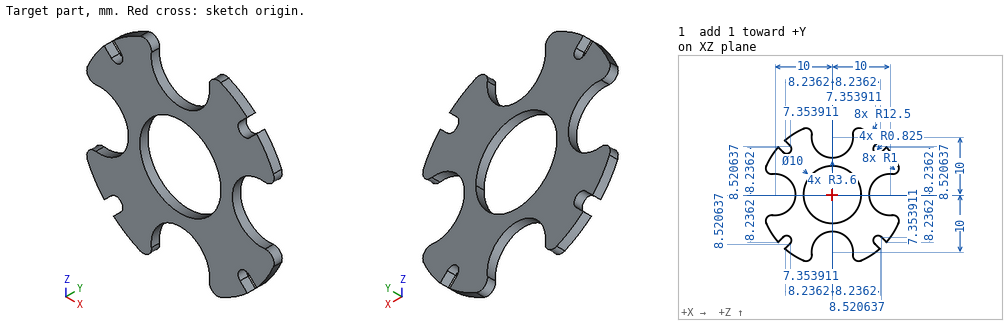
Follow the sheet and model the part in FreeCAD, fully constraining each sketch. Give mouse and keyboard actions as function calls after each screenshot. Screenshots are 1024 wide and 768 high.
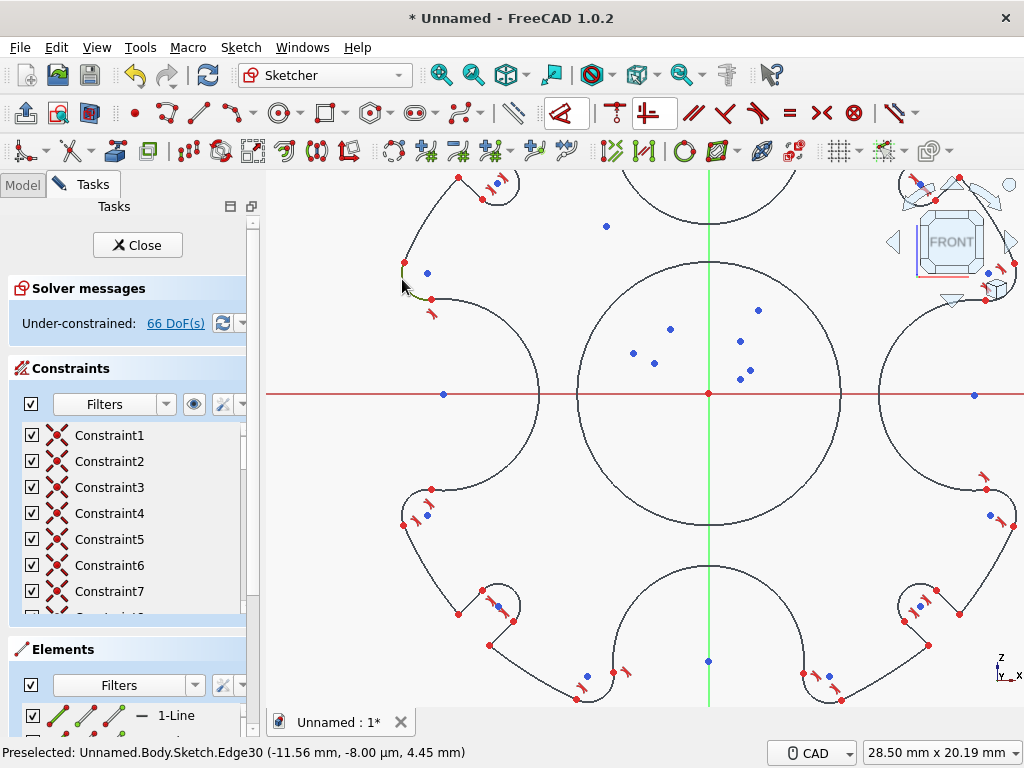
click(439, 201)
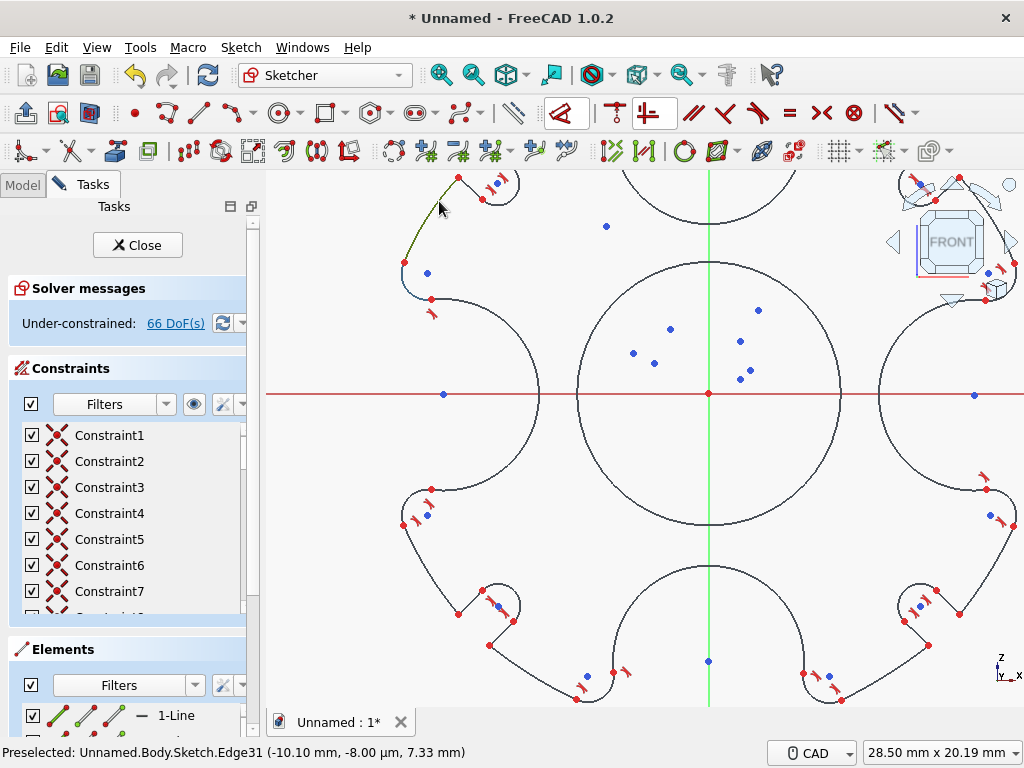
click(758, 114)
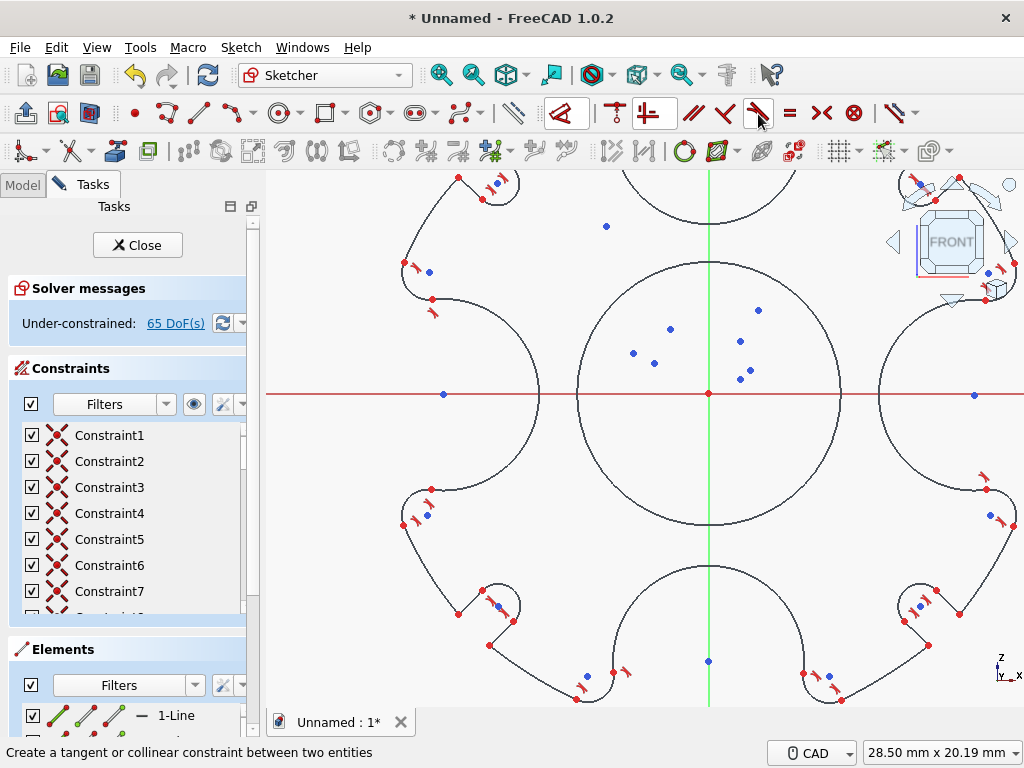
click(802, 300)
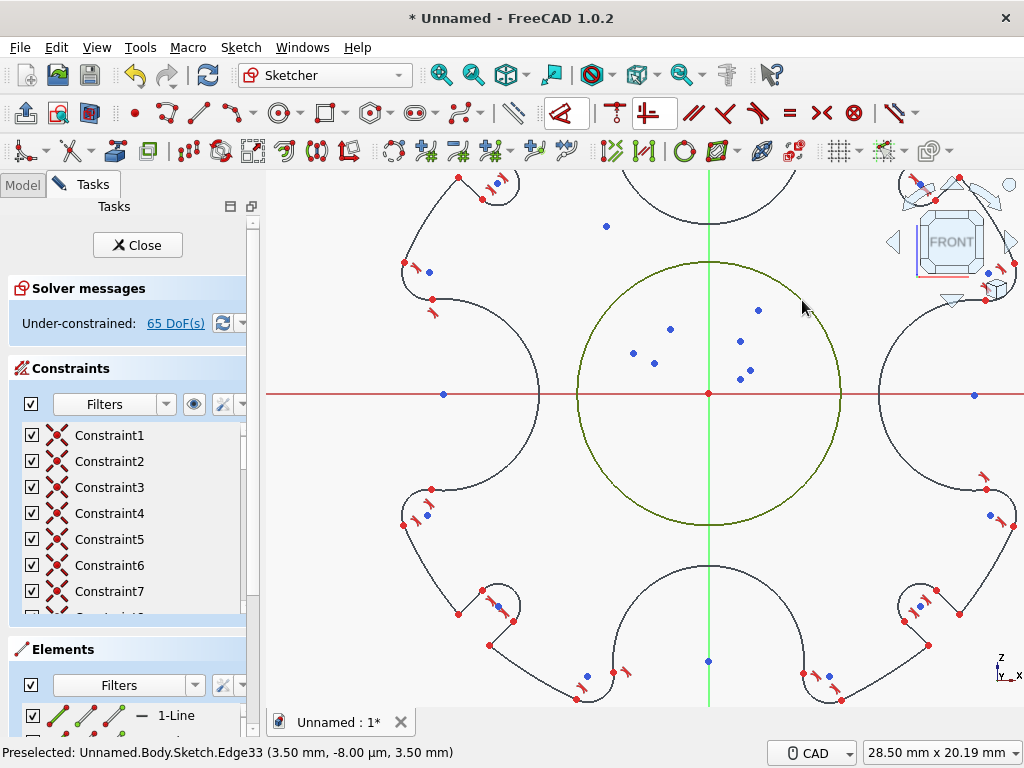
scroll(415, 493, down, 3)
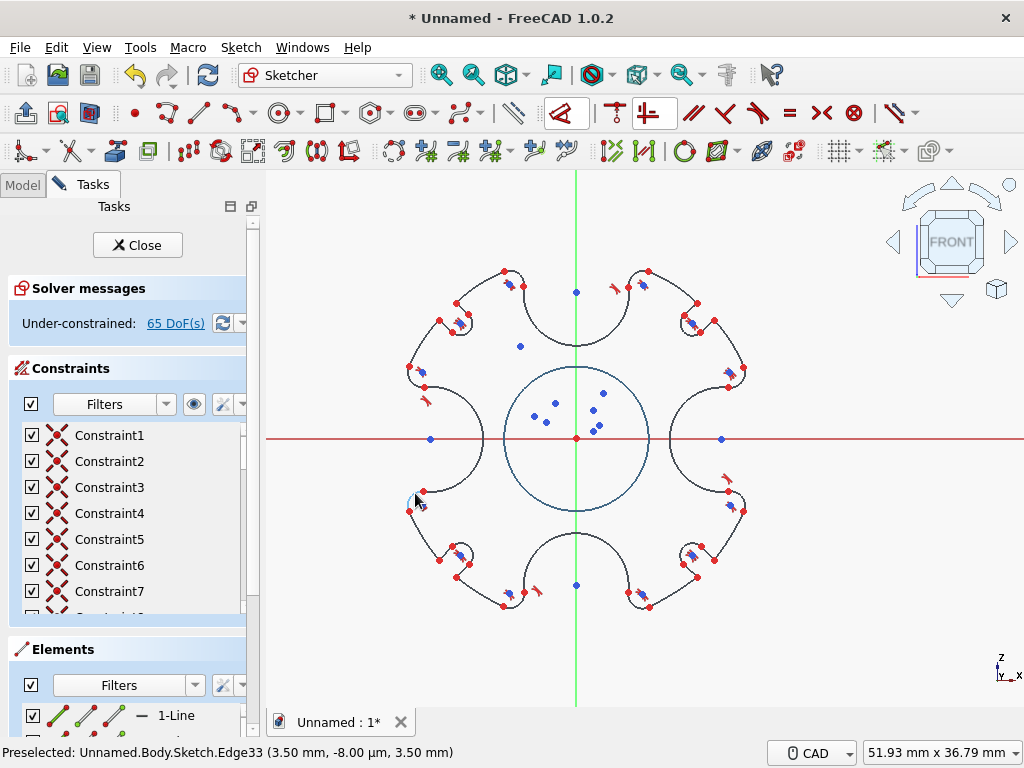
click(489, 279)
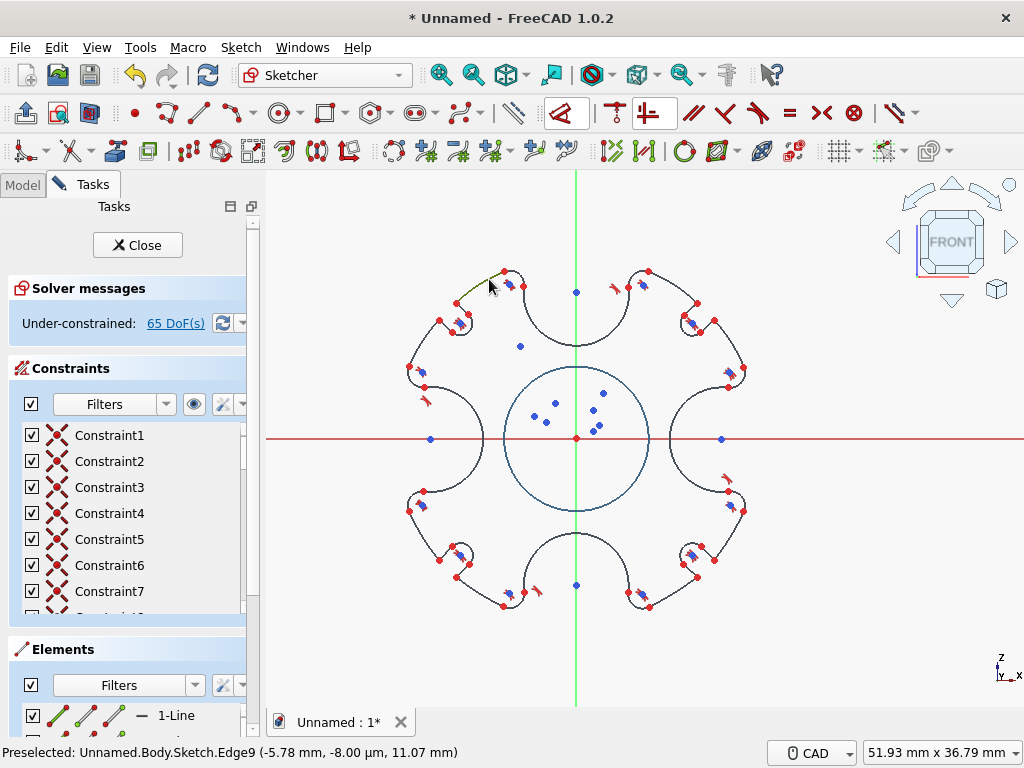
click(616, 114)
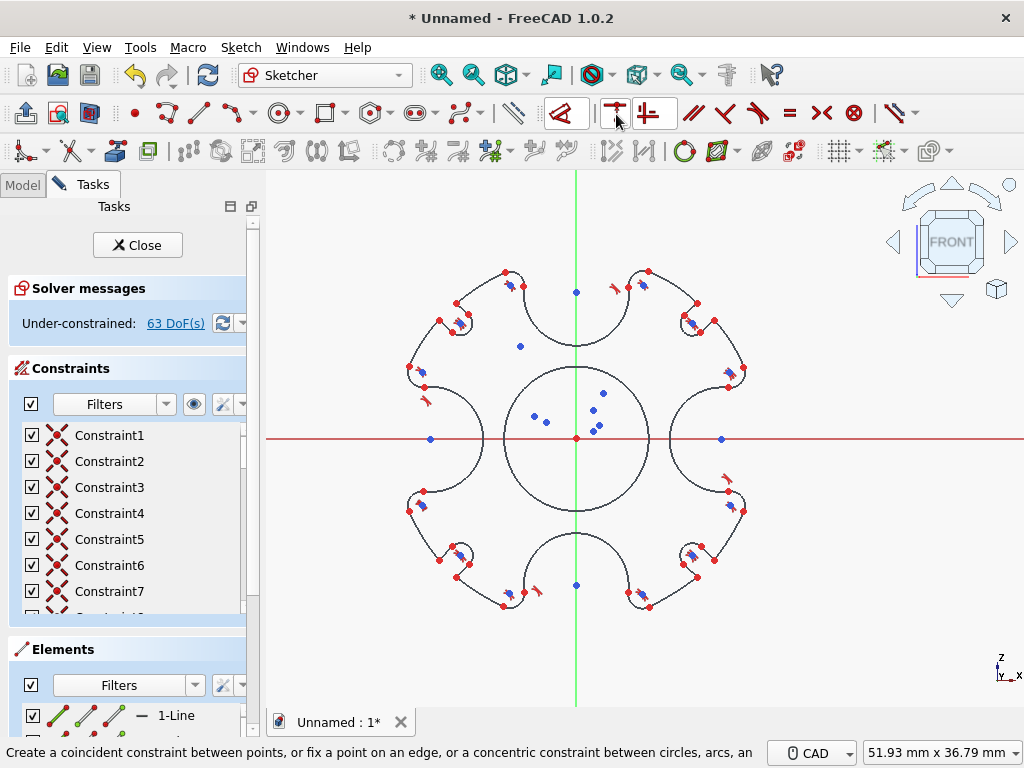
click(627, 387)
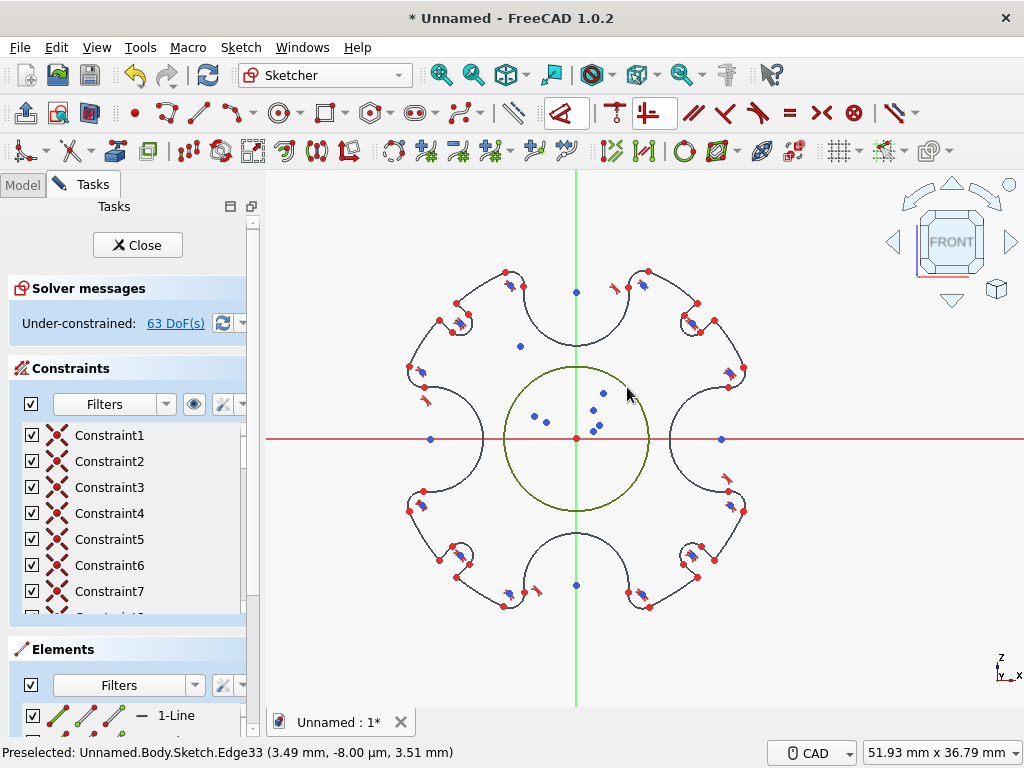
click(684, 292)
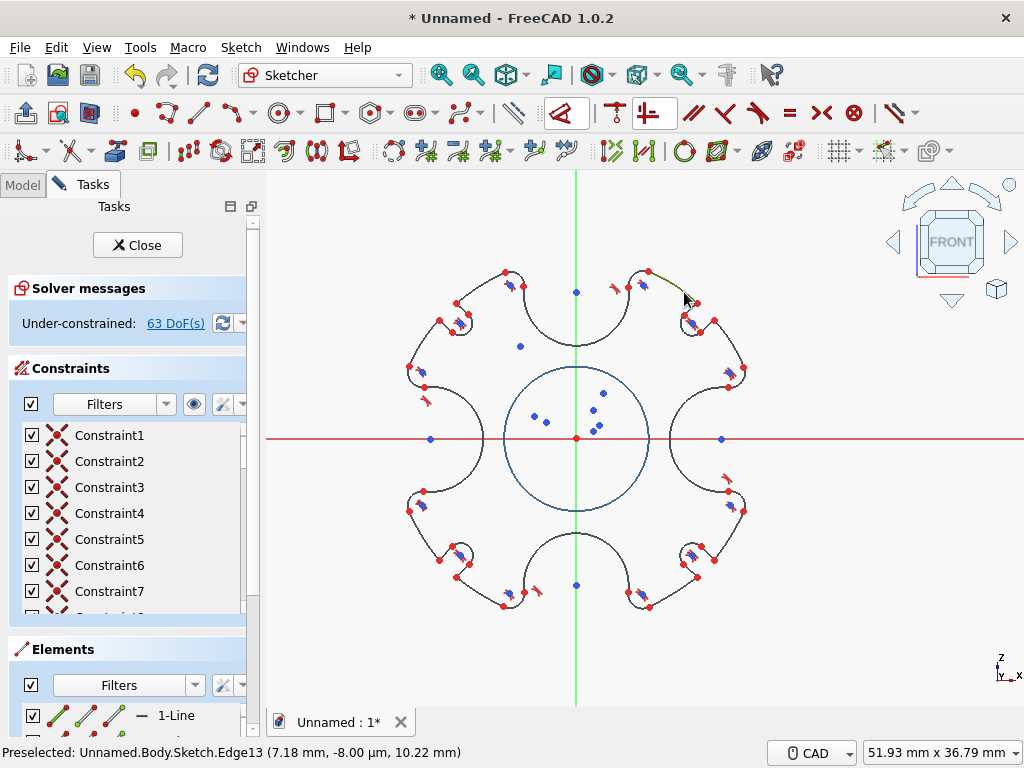
click(616, 114)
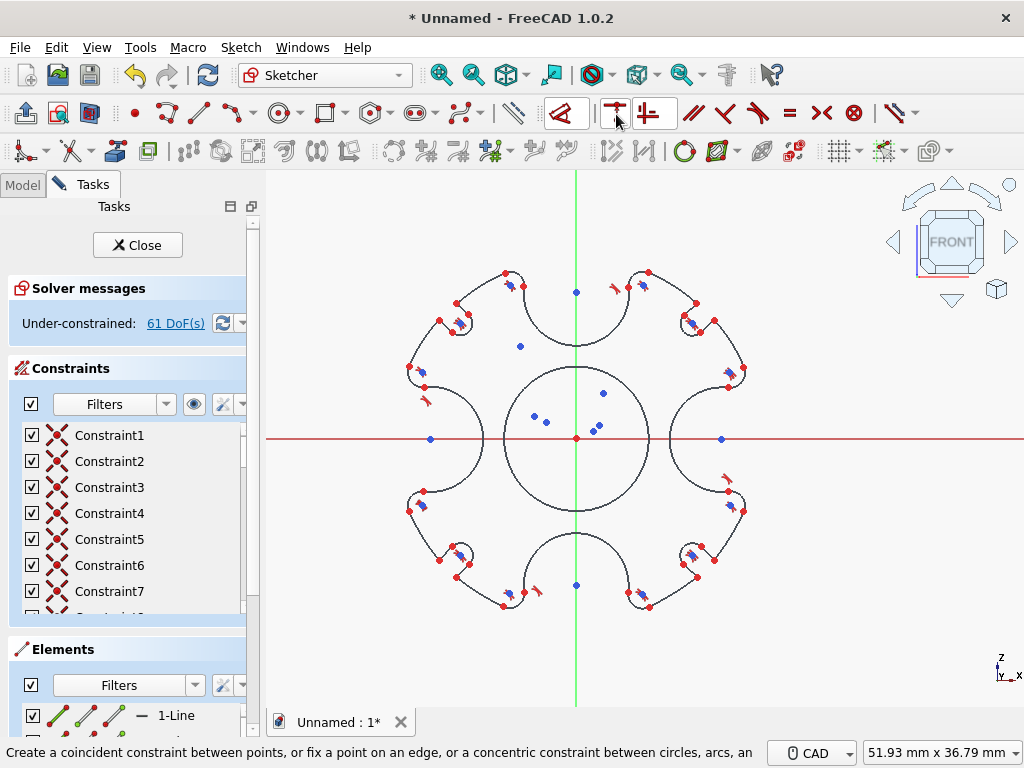
click(627, 387)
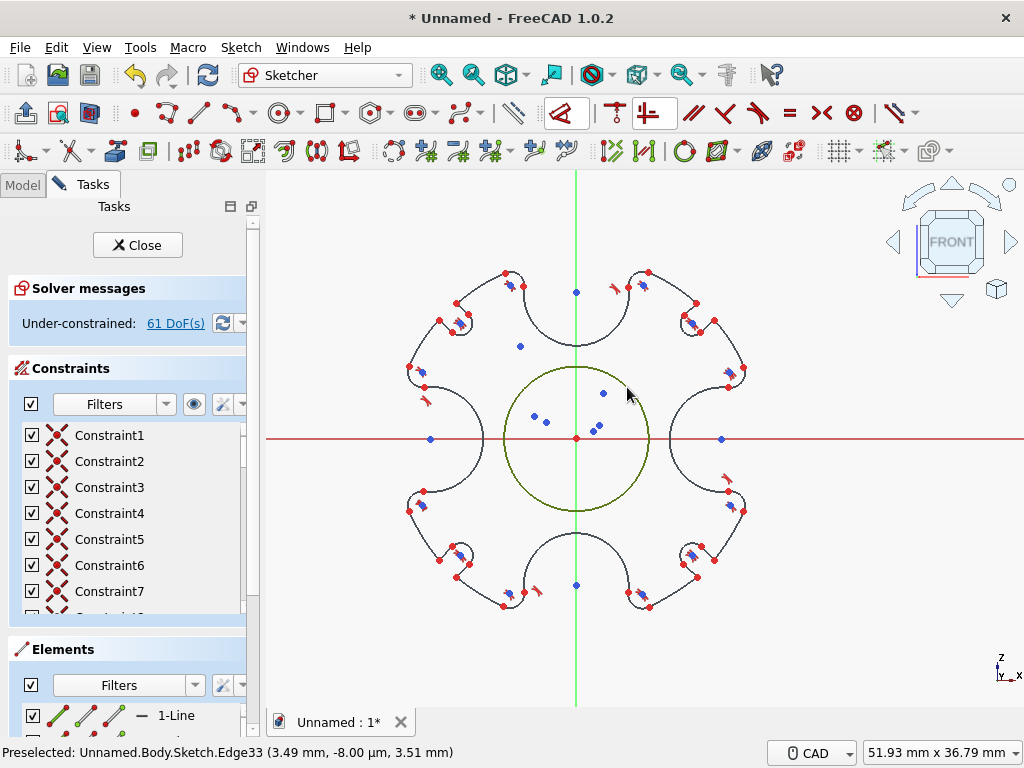
click(737, 352)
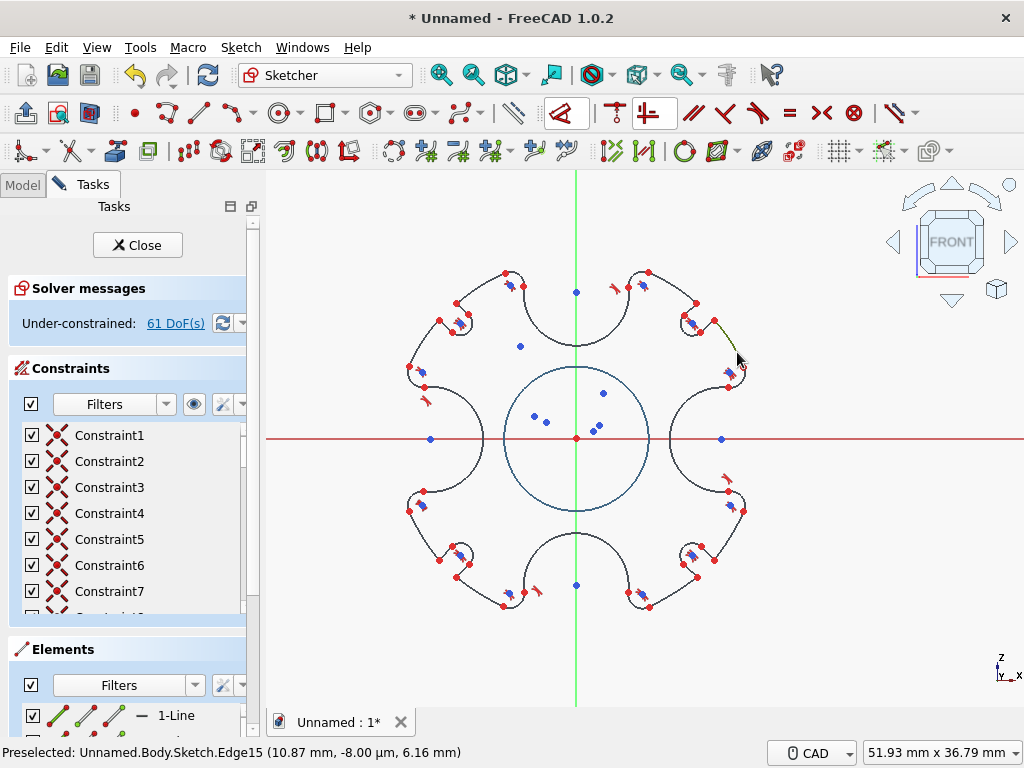
key(c)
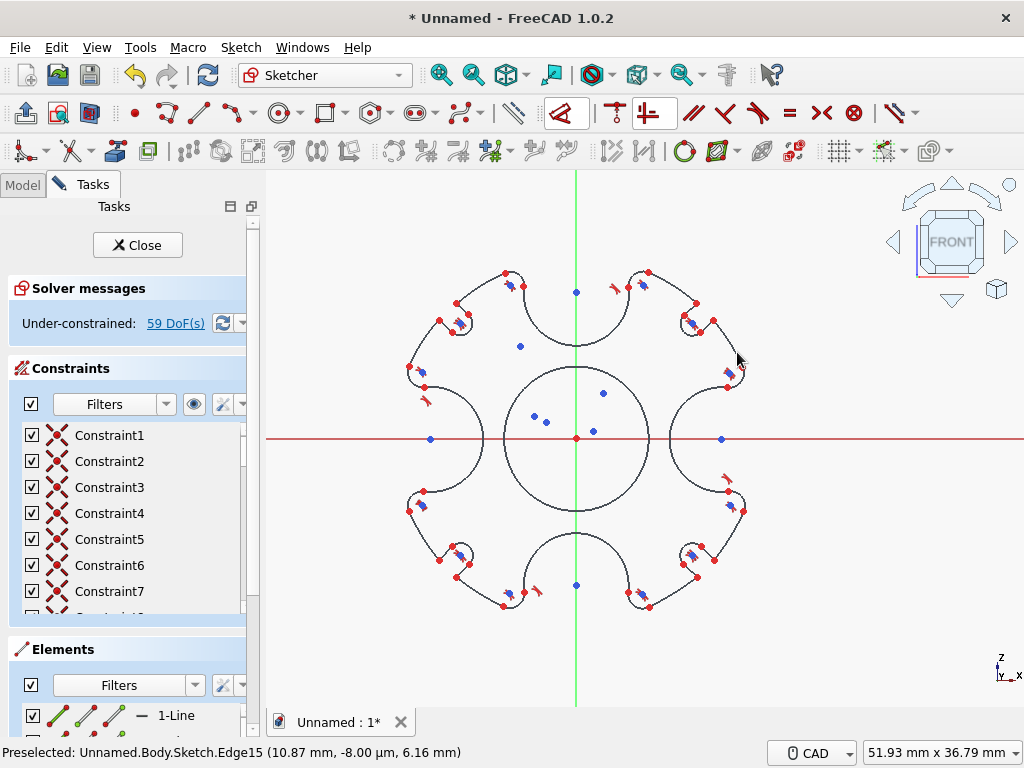
click(627, 387)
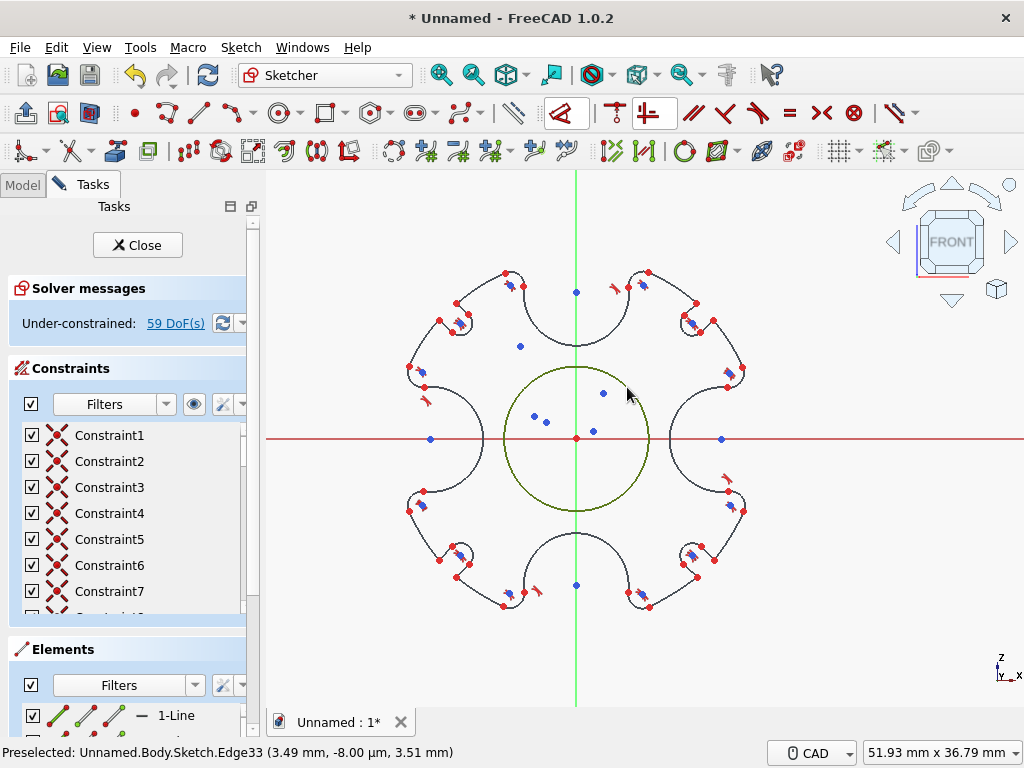
click(724, 546)